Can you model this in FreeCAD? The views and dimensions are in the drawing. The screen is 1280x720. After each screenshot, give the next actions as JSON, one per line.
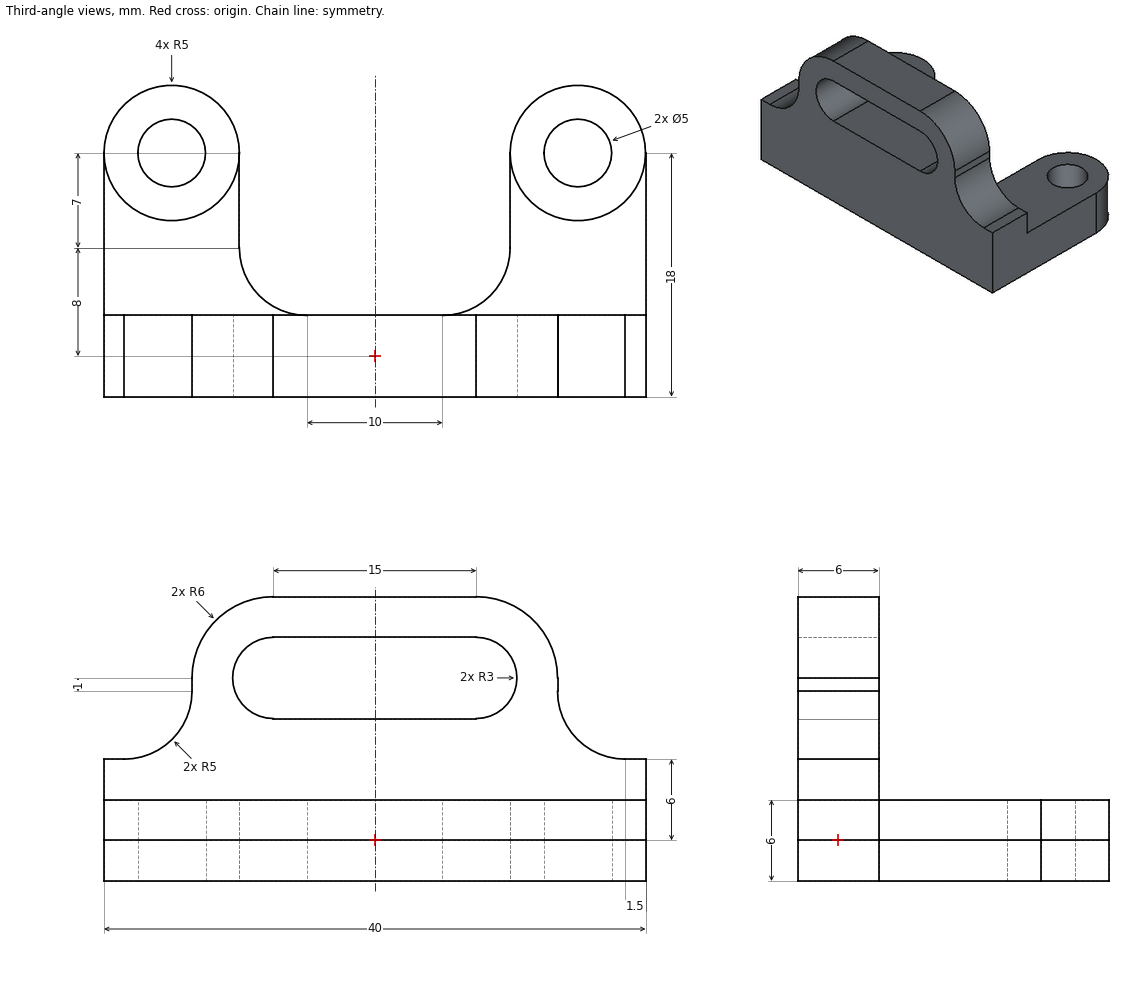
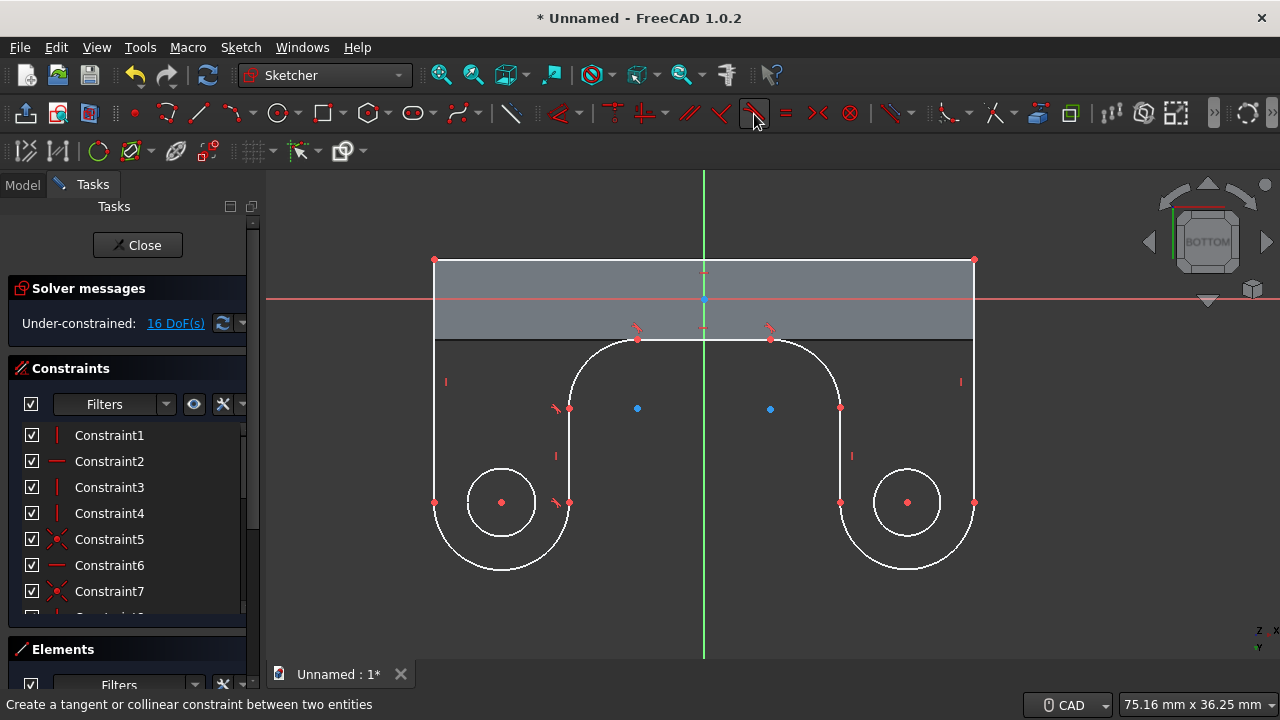
{"action": "left_click", "coordinate": [840, 436]}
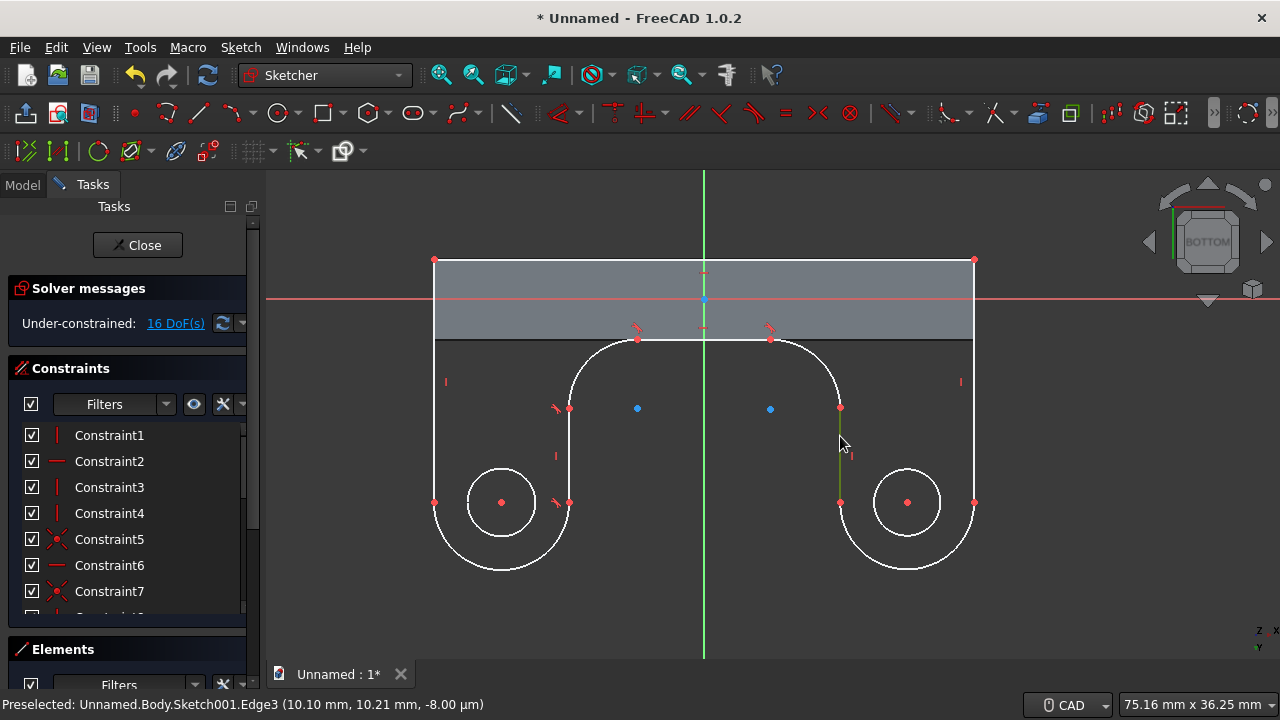
{"action": "left_click", "coordinate": [832, 377]}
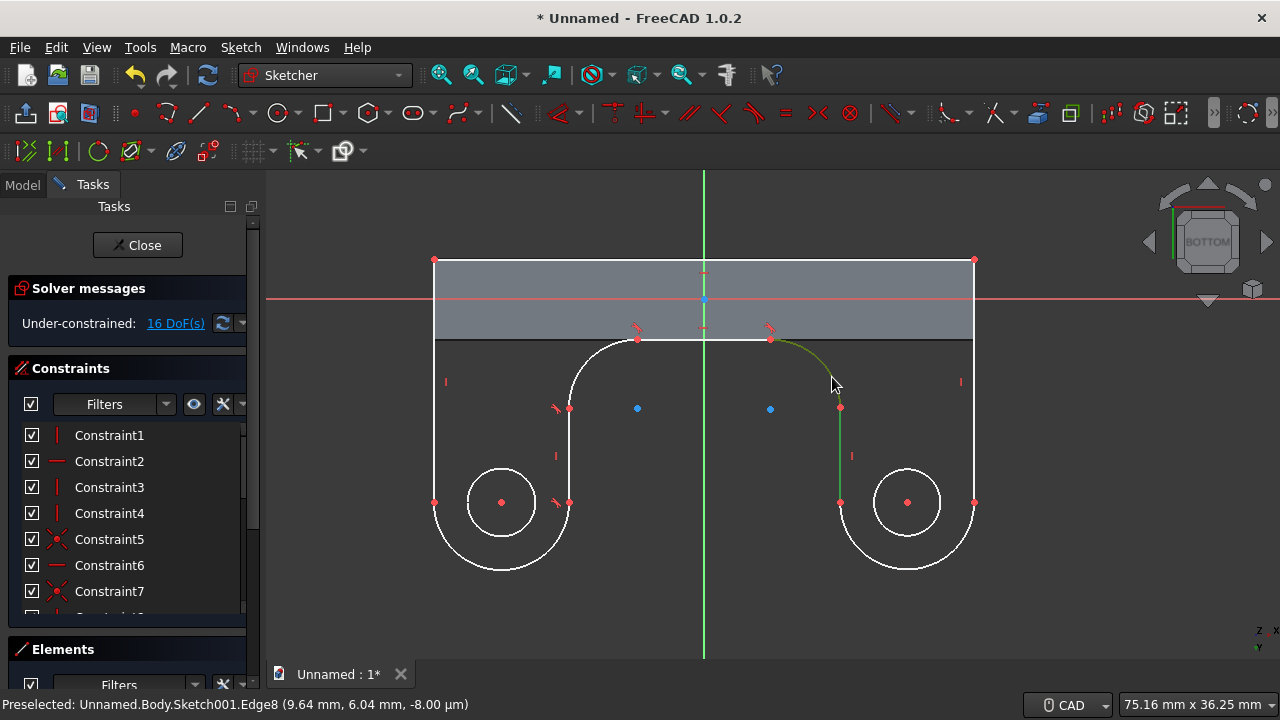
{"action": "left_click", "coordinate": [754, 114]}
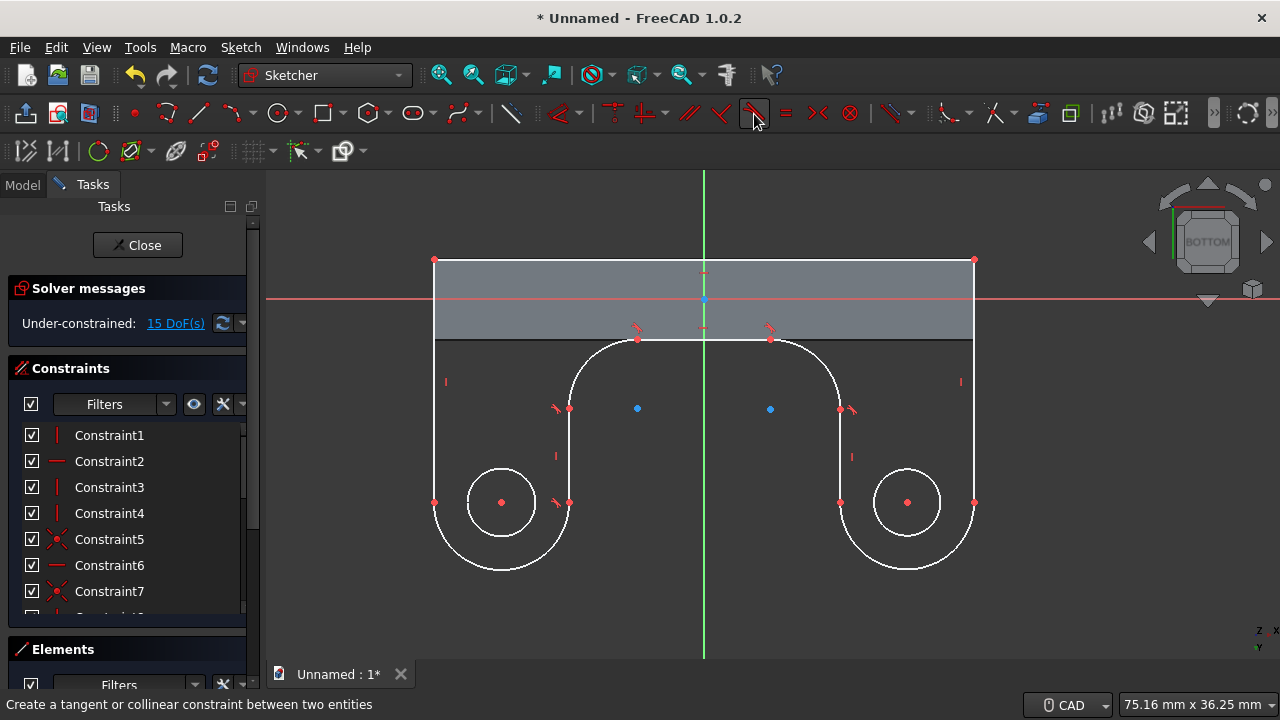
{"action": "left_click", "coordinate": [840, 437]}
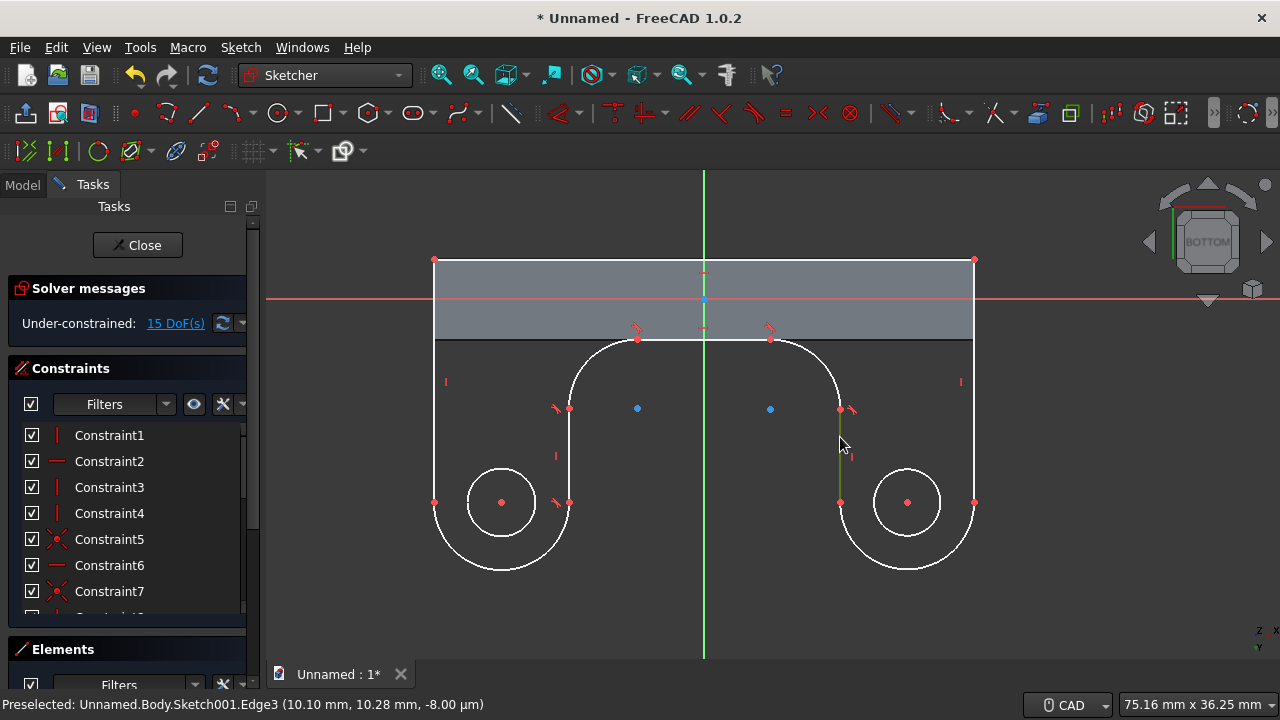
{"action": "left_click", "coordinate": [868, 557]}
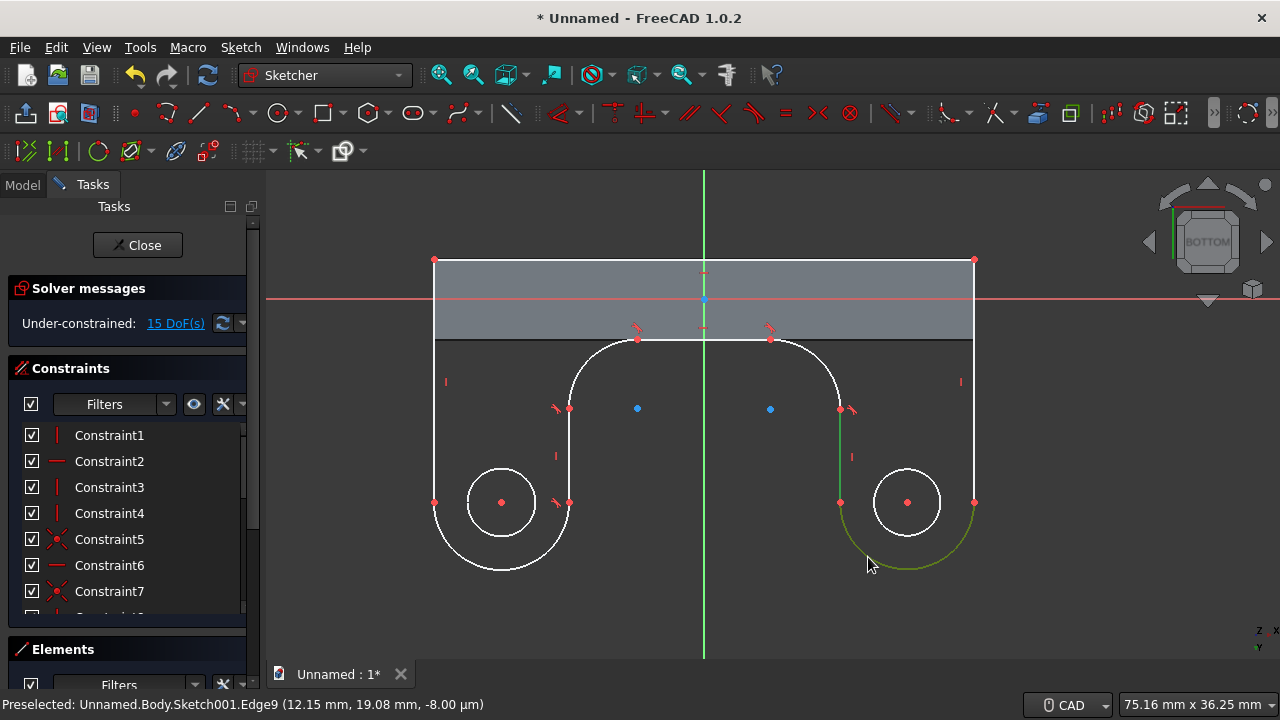
{"action": "left_click", "coordinate": [754, 114]}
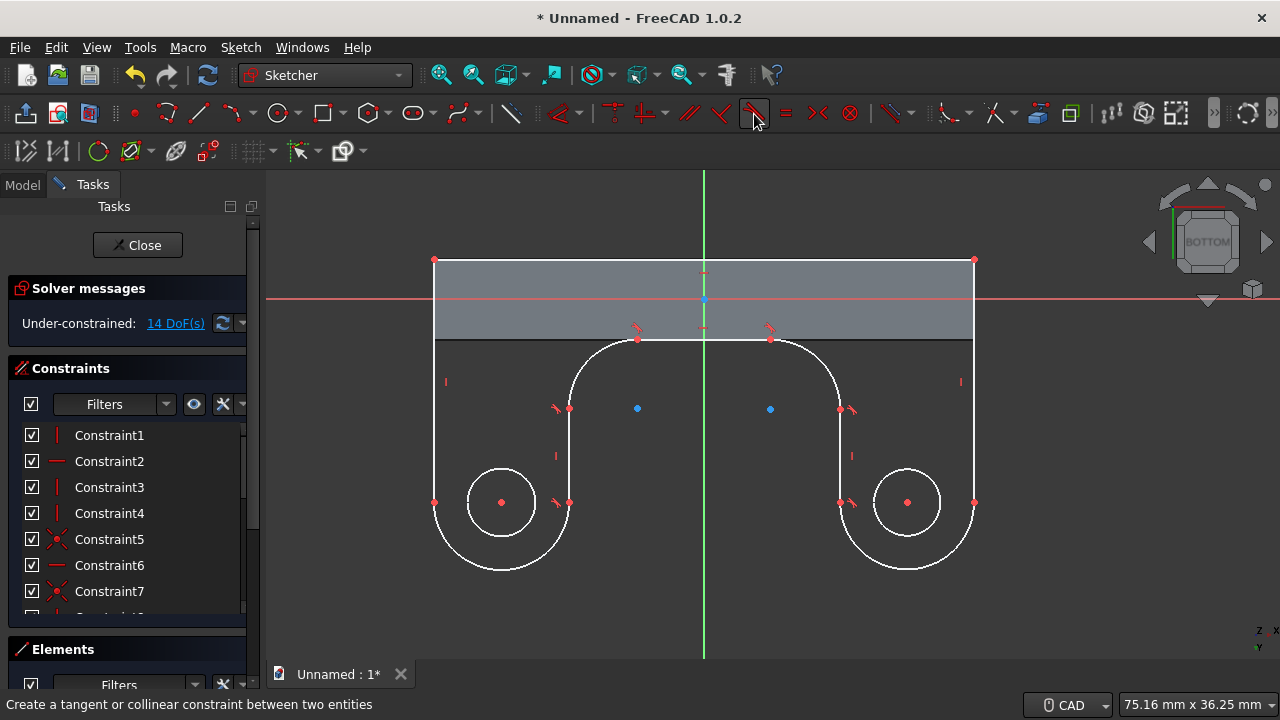
{"action": "left_click", "coordinate": [974, 430]}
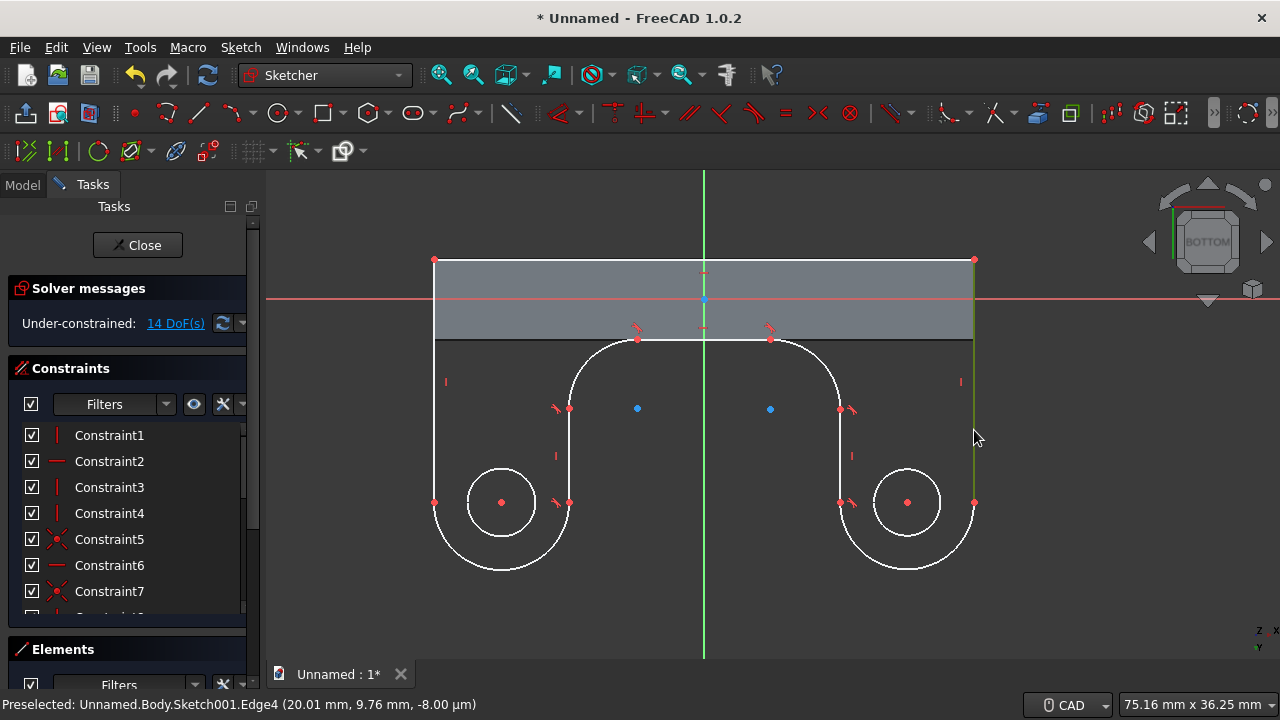
{"action": "left_click", "coordinate": [868, 557]}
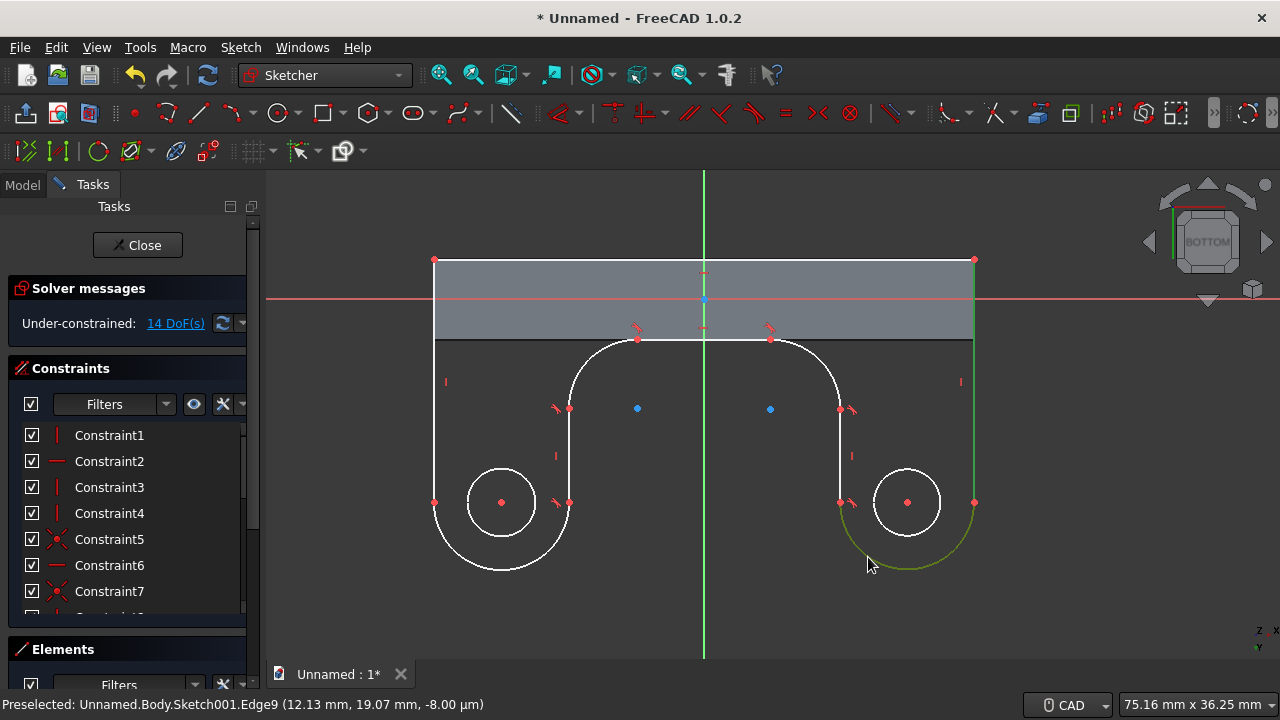
{"action": "left_click", "coordinate": [754, 114]}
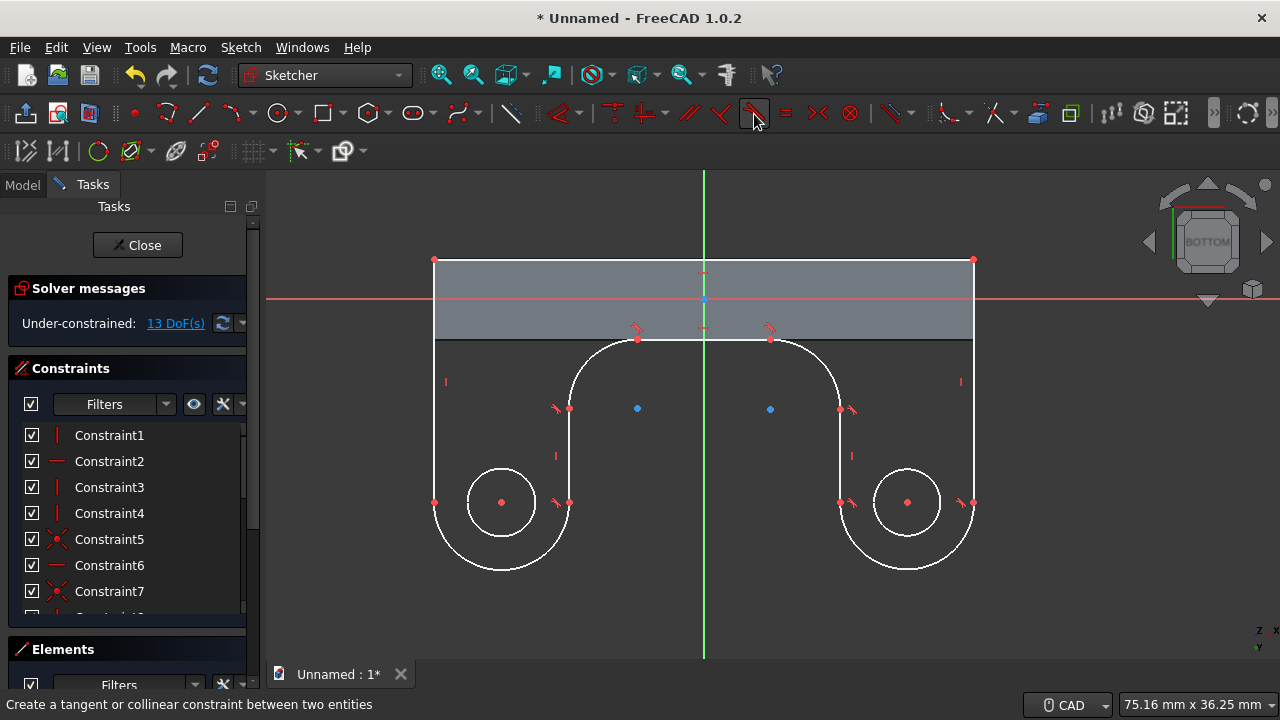
{"action": "left_click", "coordinate": [434, 333]}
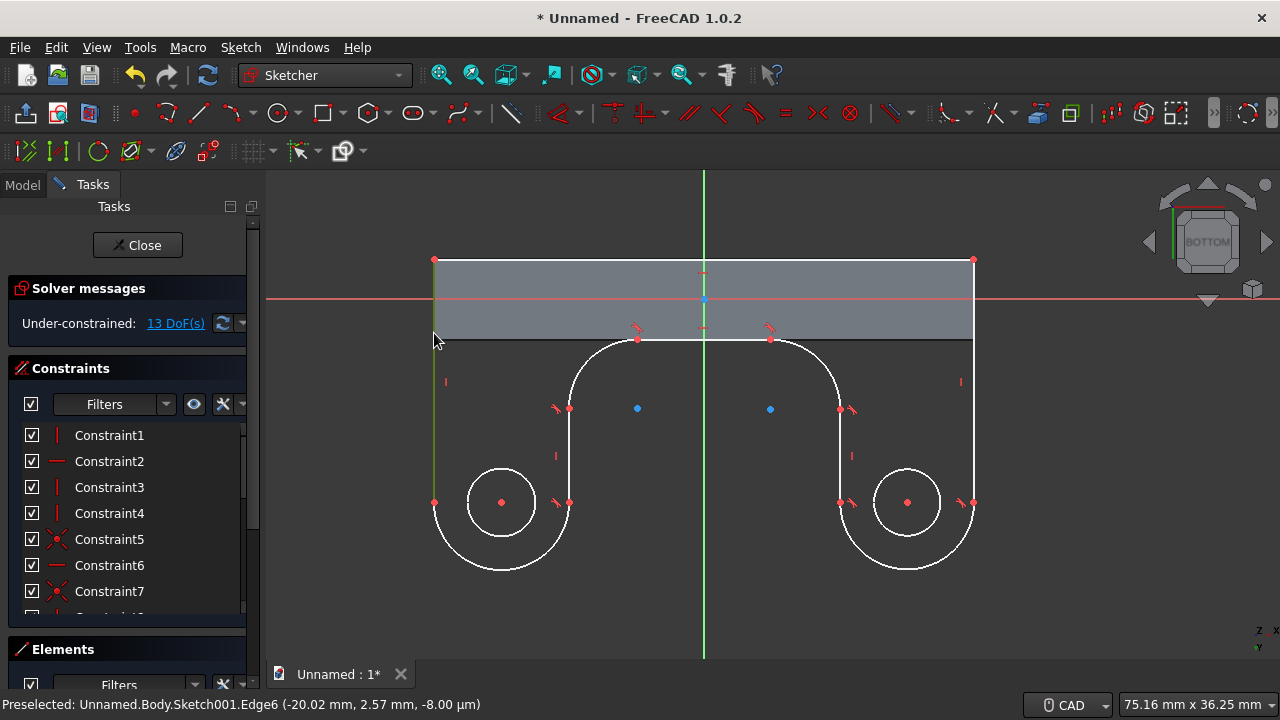
{"action": "left_click", "coordinate": [462, 557]}